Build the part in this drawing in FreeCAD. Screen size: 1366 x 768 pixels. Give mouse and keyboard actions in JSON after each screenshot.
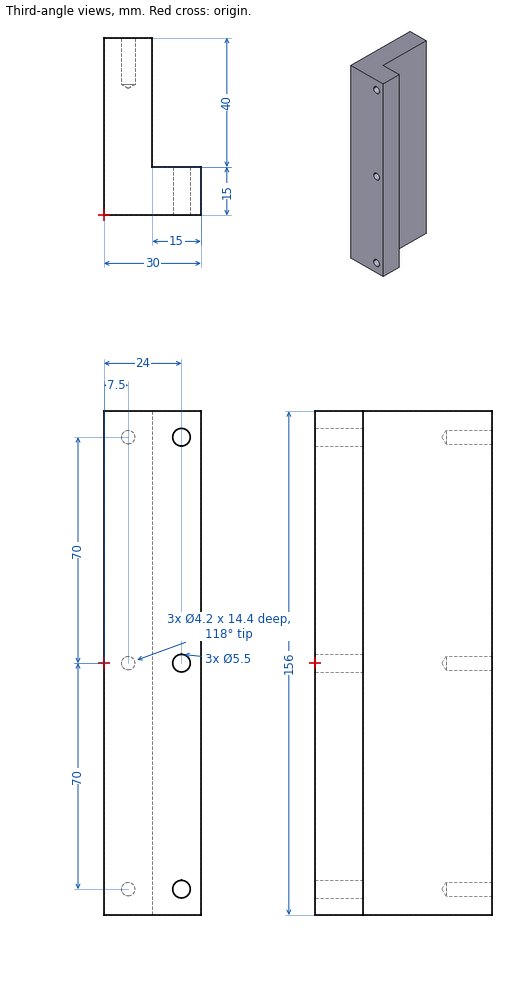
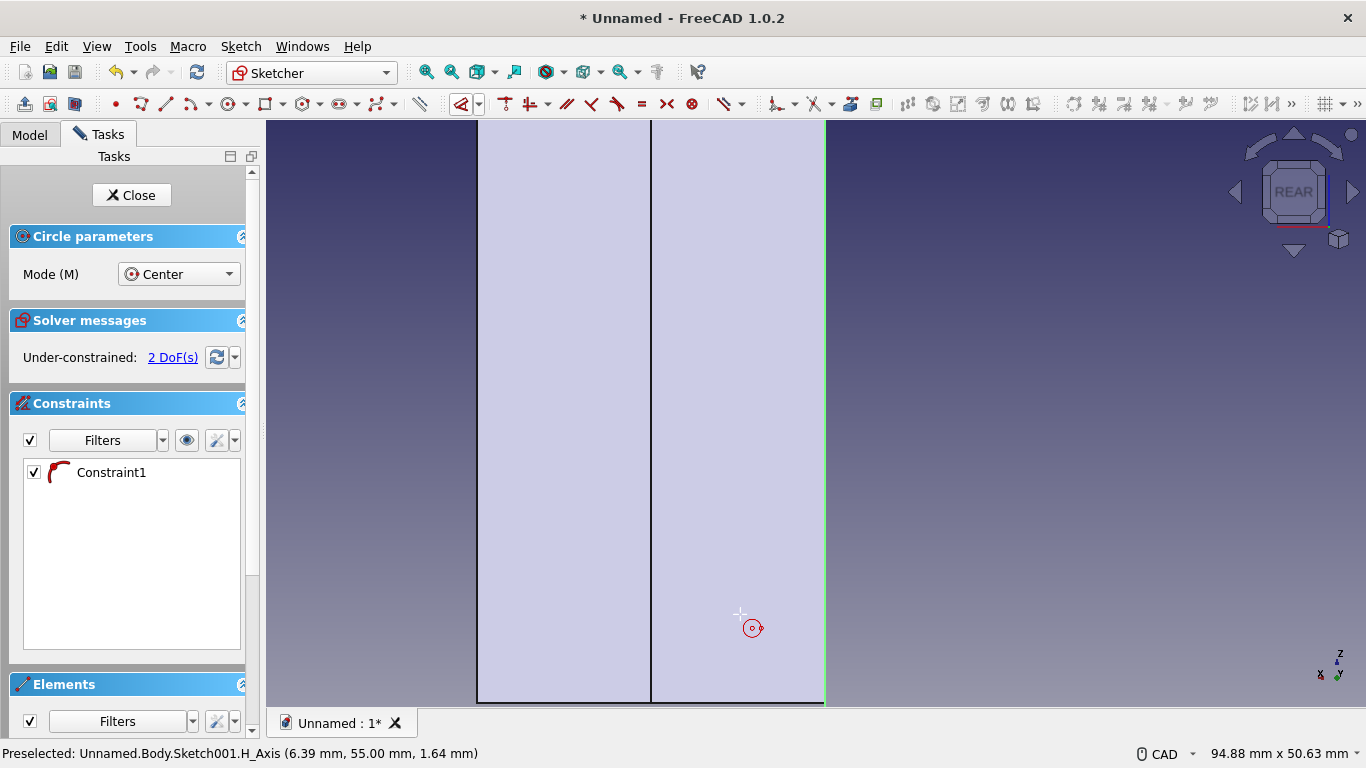
{"action": "scroll", "coordinate": [740, 615], "scroll_direction": "down", "scroll_amount": 7}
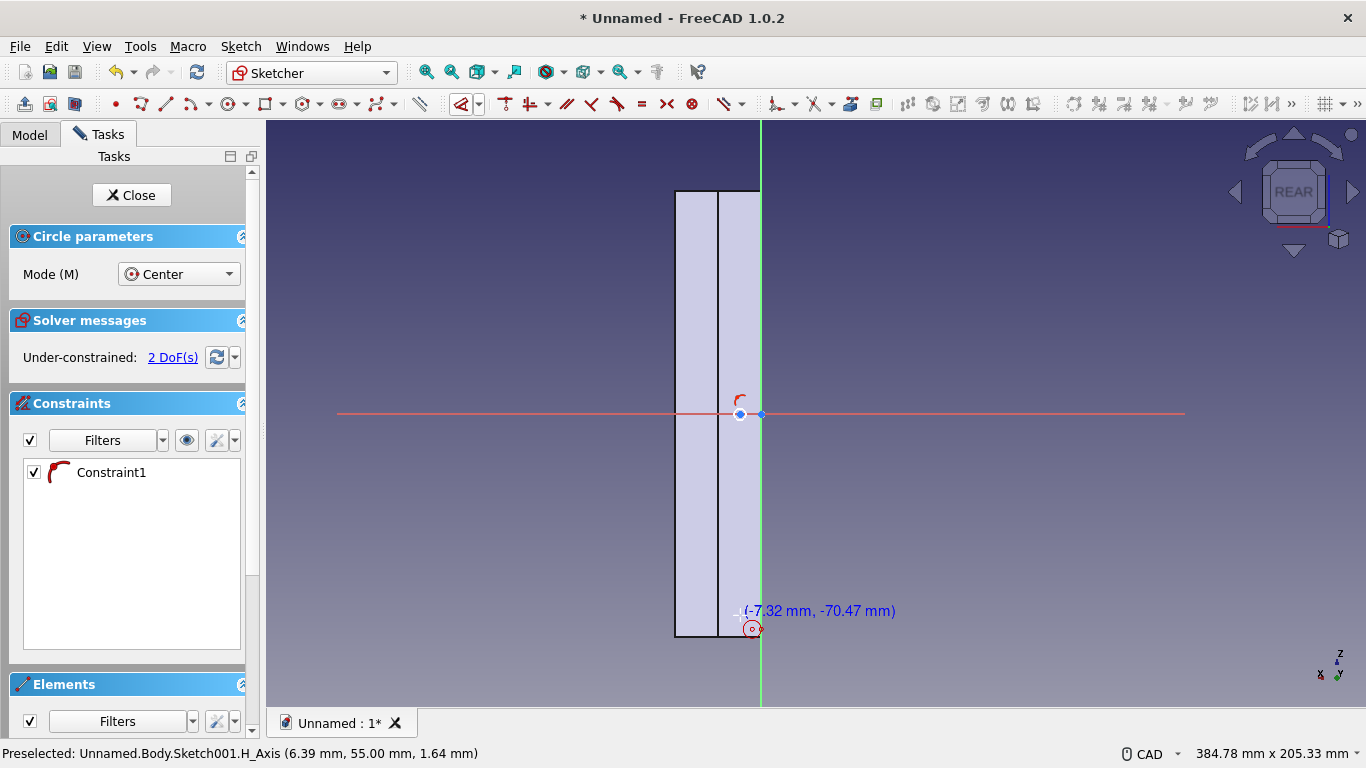
{"action": "left_click", "coordinate": [740, 615]}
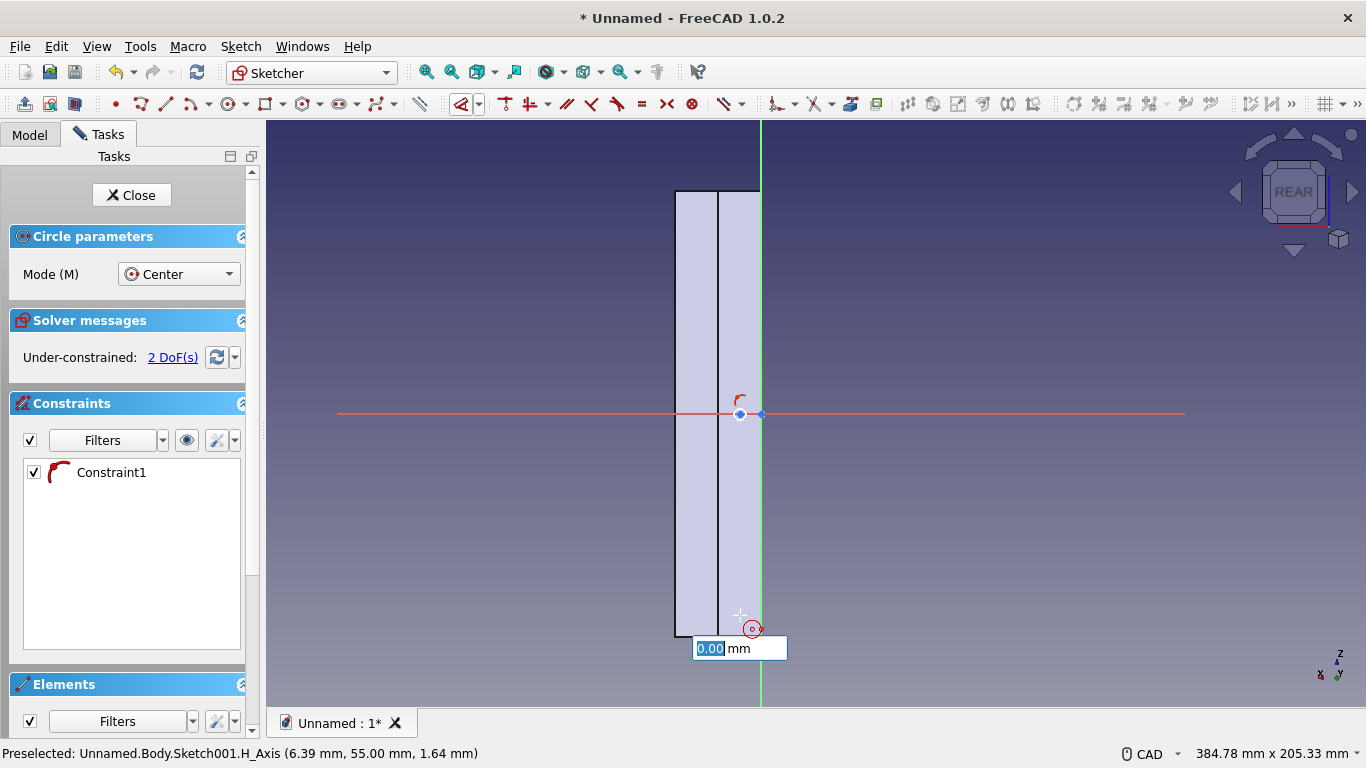
{"action": "scroll", "coordinate": [744, 610], "scroll_direction": "up", "scroll_amount": 5}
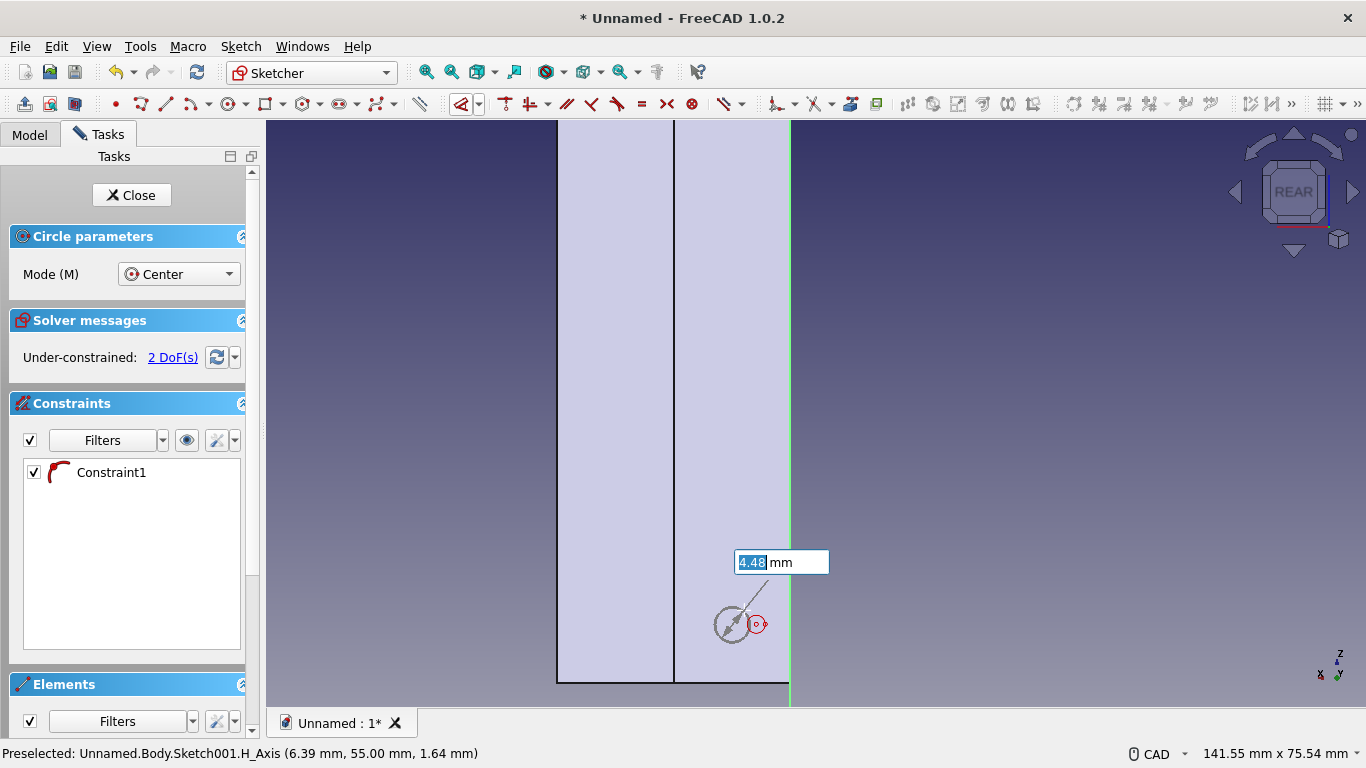
{"action": "left_click", "coordinate": [743, 609]}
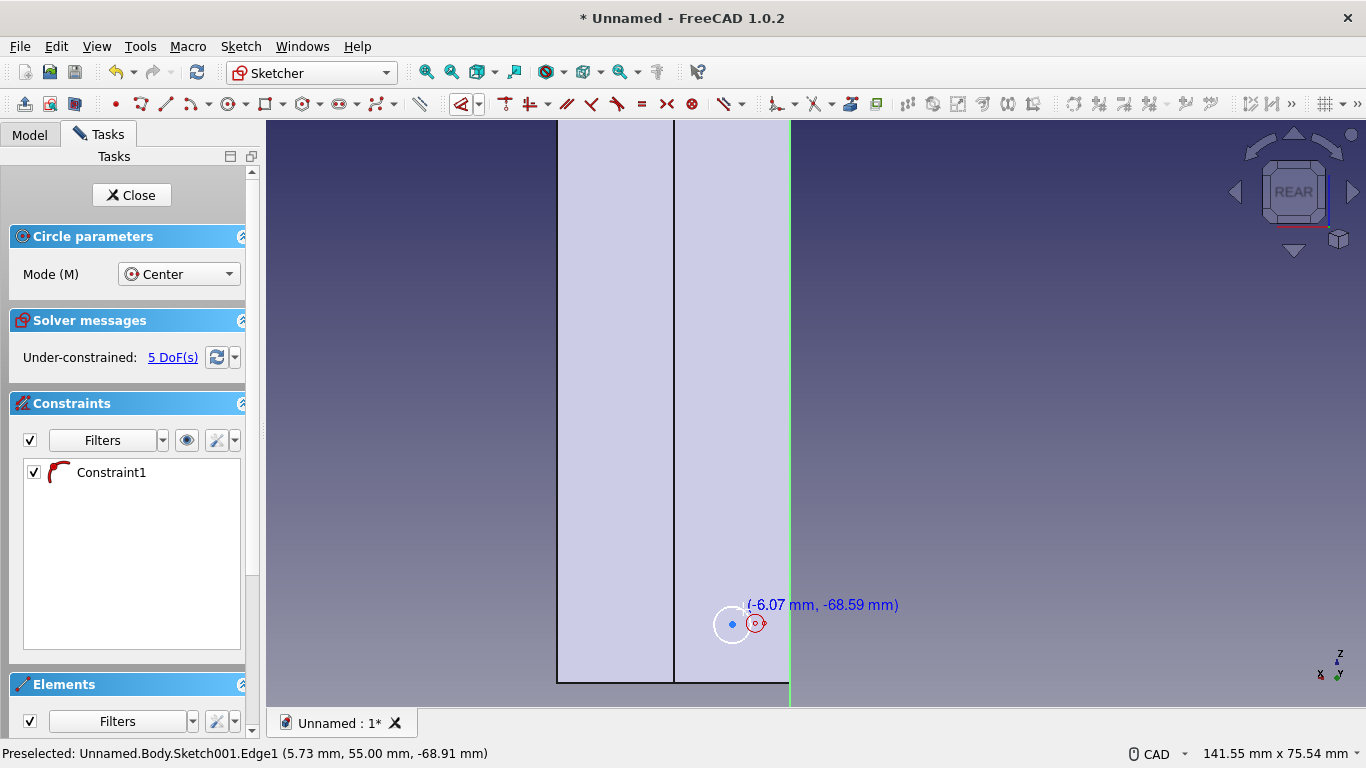
{"action": "scroll", "coordinate": [744, 609], "scroll_direction": "down", "scroll_amount": 5}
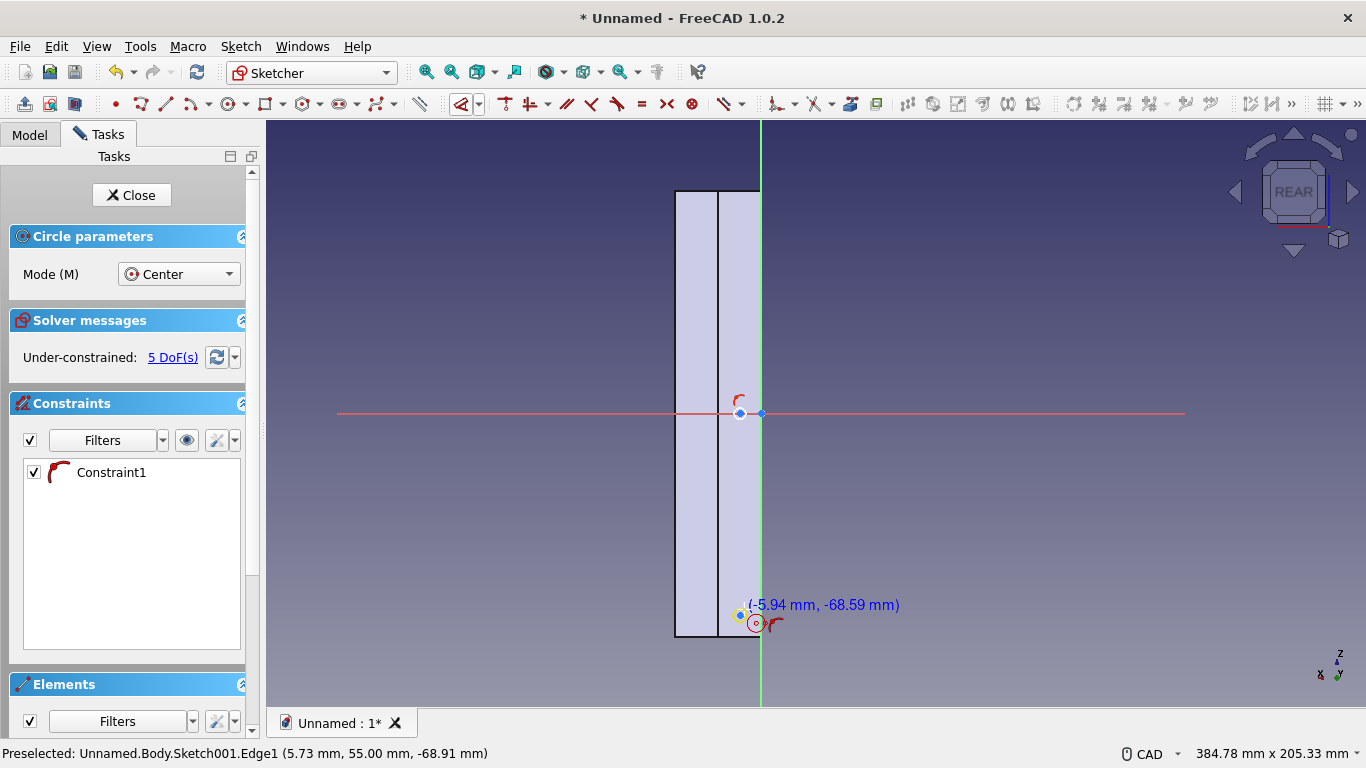
{"action": "scroll", "coordinate": [740, 214], "scroll_direction": "up", "scroll_amount": 7}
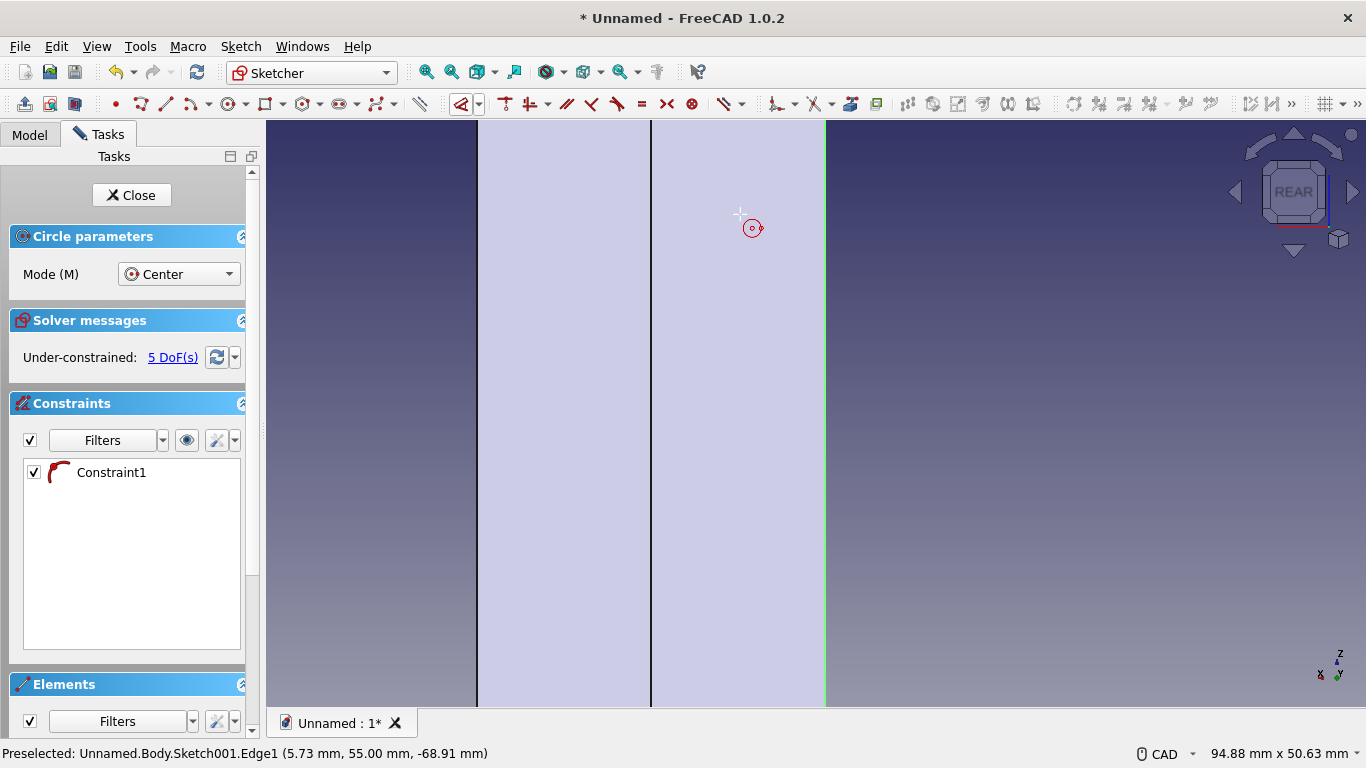
{"action": "scroll", "coordinate": [740, 214], "scroll_direction": "down", "scroll_amount": 7}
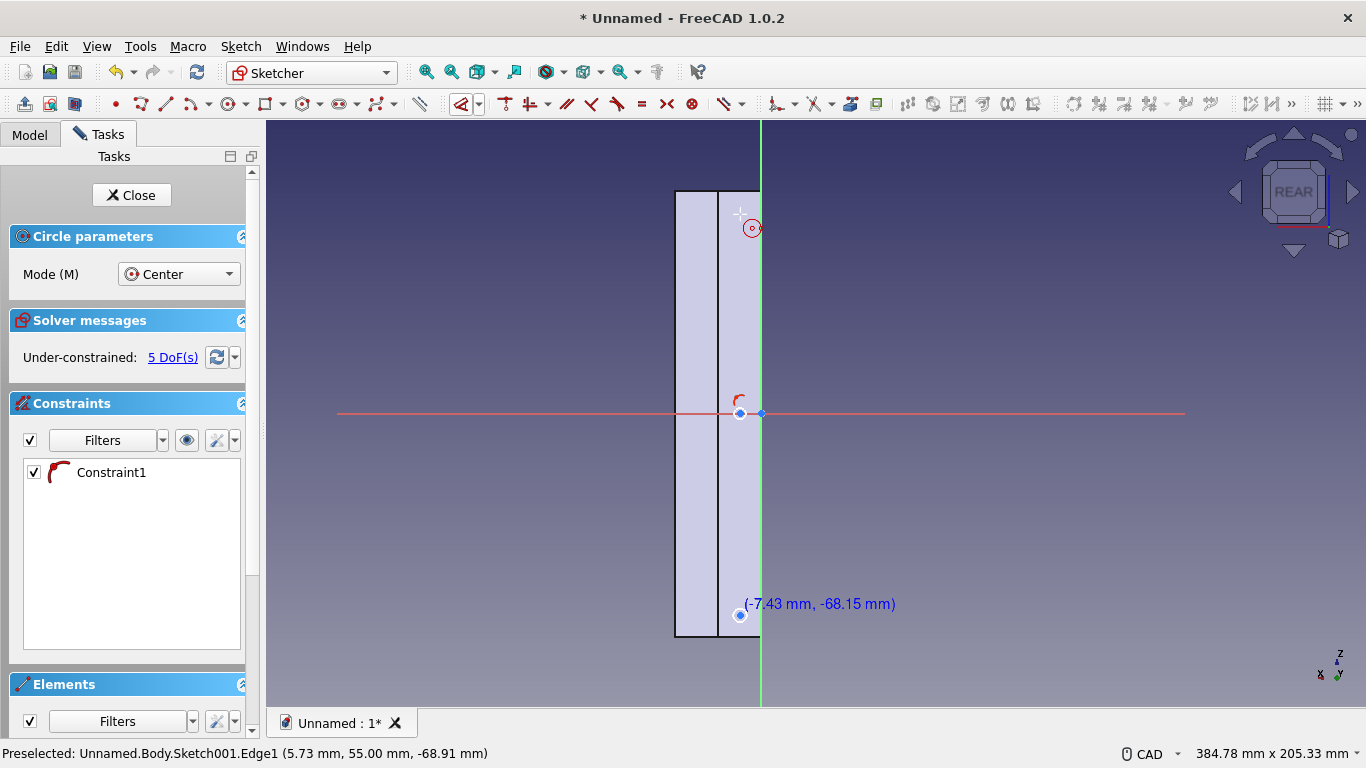
{"action": "left_click", "coordinate": [740, 214]}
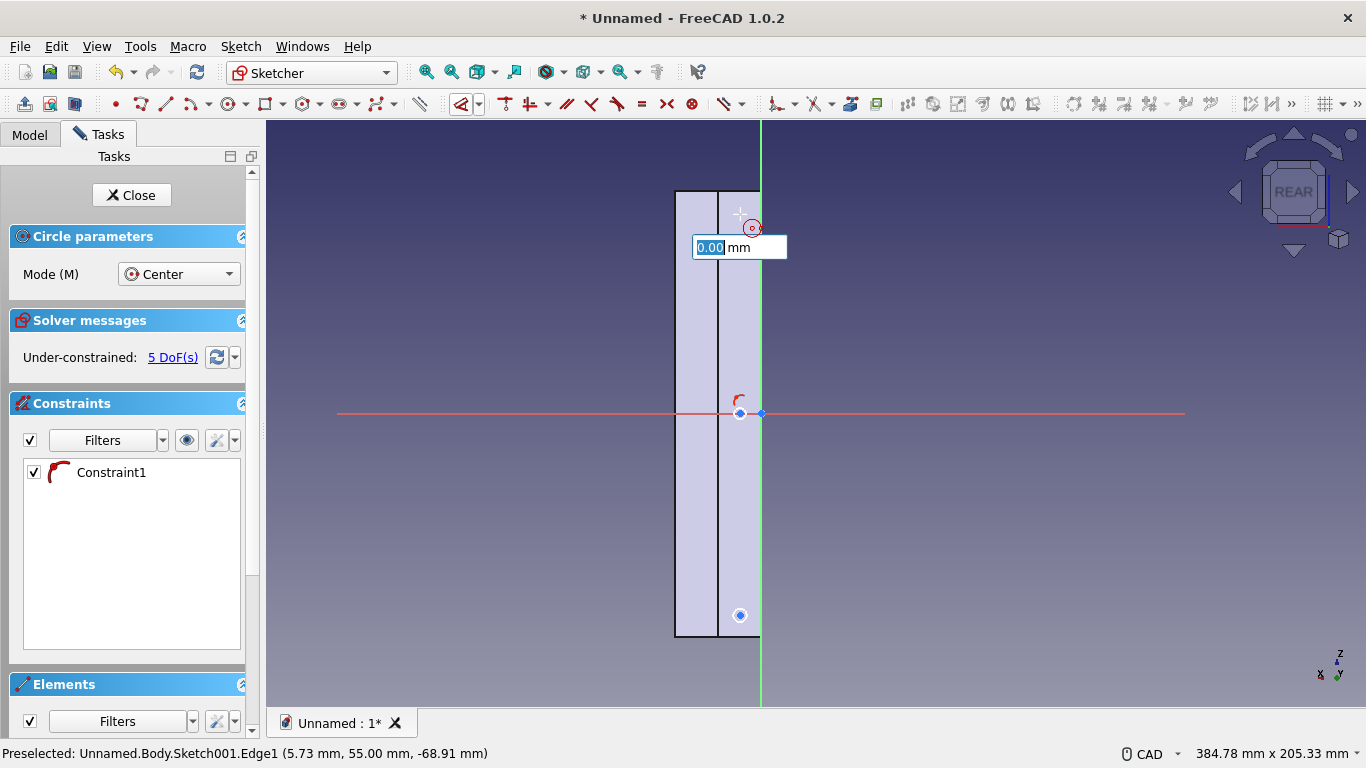
{"action": "scroll", "coordinate": [744, 209], "scroll_direction": "up", "scroll_amount": 5}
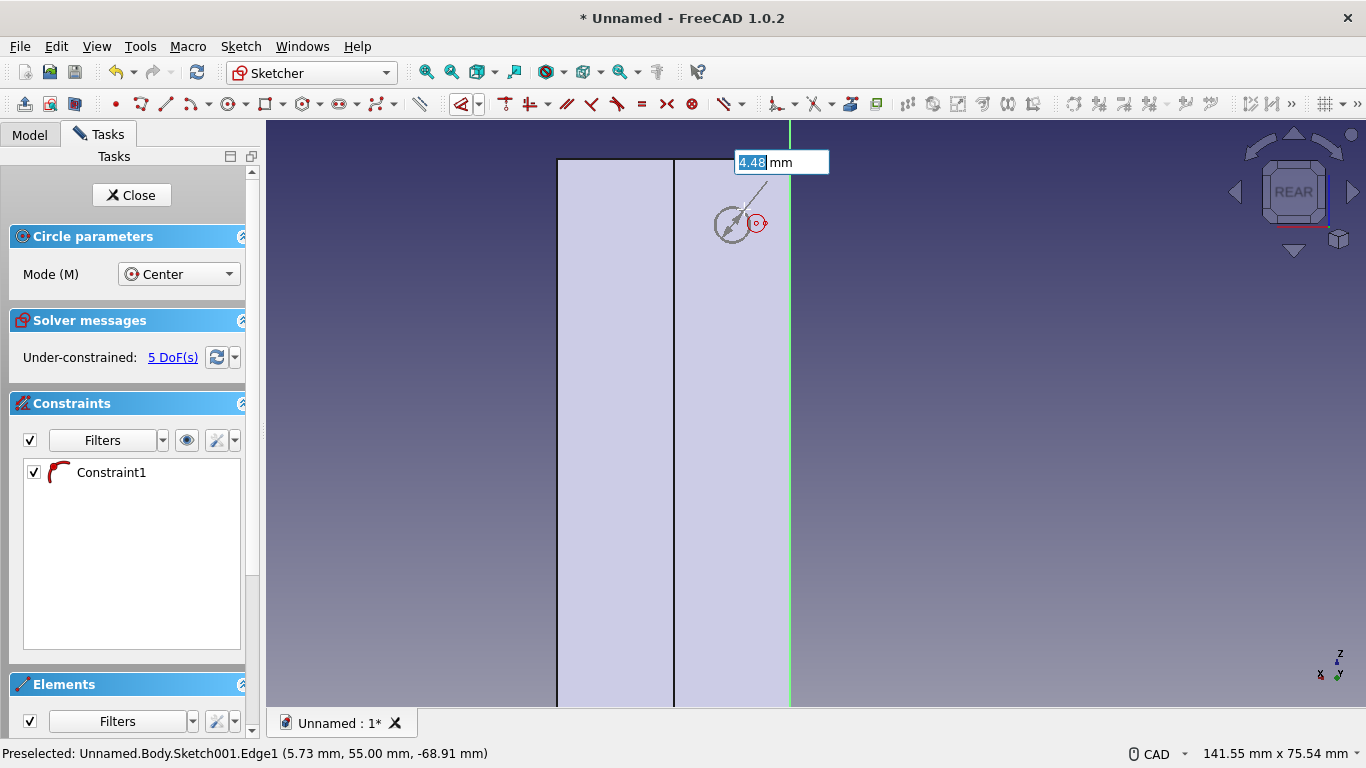
{"action": "left_click", "coordinate": [743, 210]}
{"action": "key", "text": "Escape"}